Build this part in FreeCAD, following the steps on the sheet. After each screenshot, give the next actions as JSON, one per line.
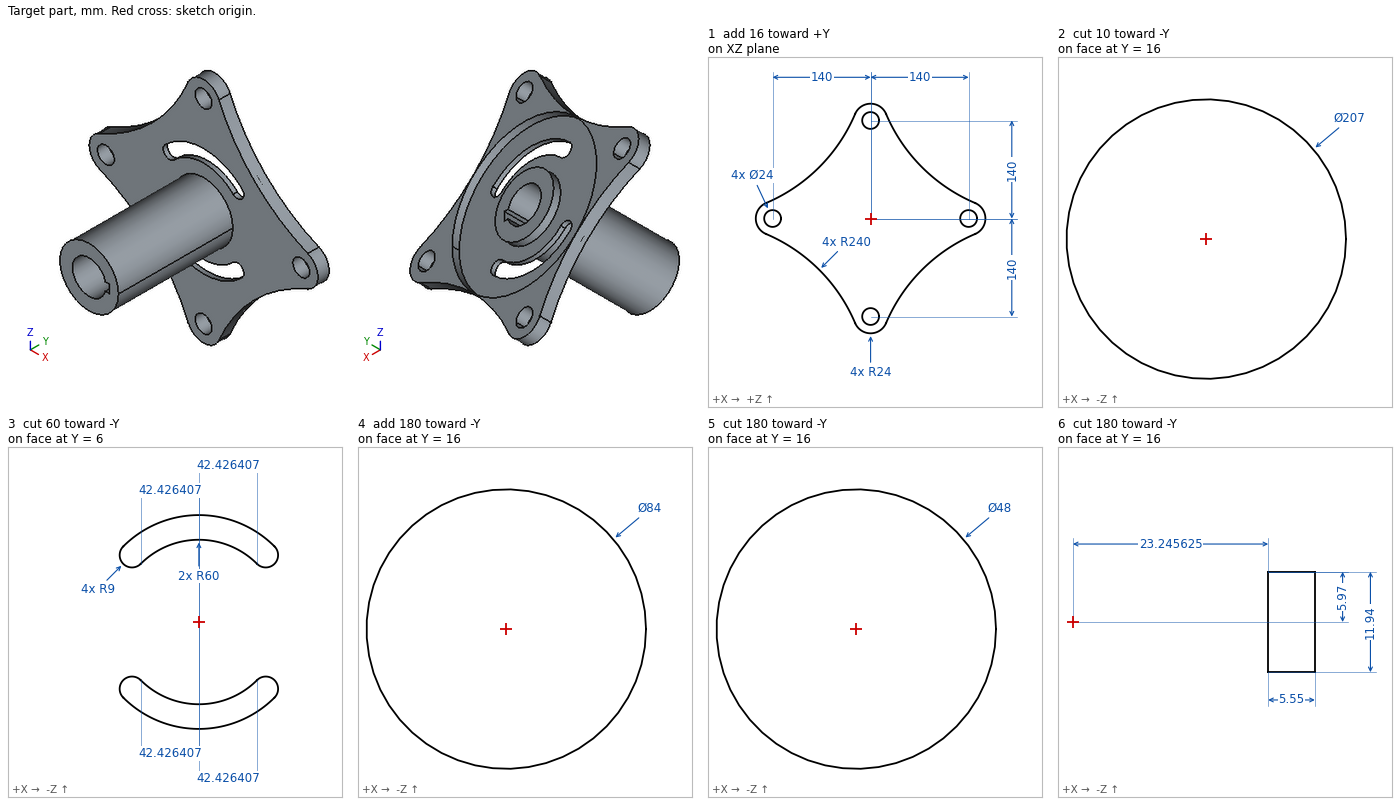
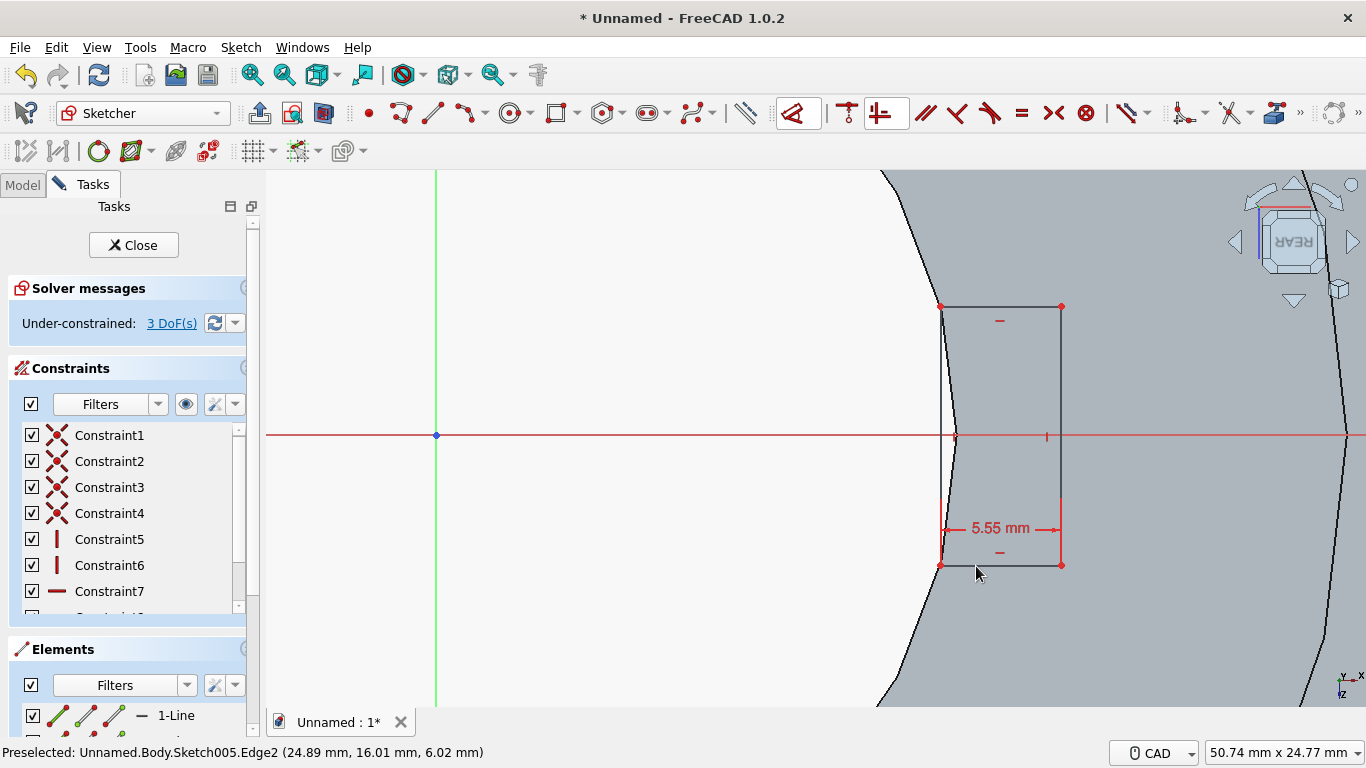
{"action": "left_click", "coordinate": [941, 385]}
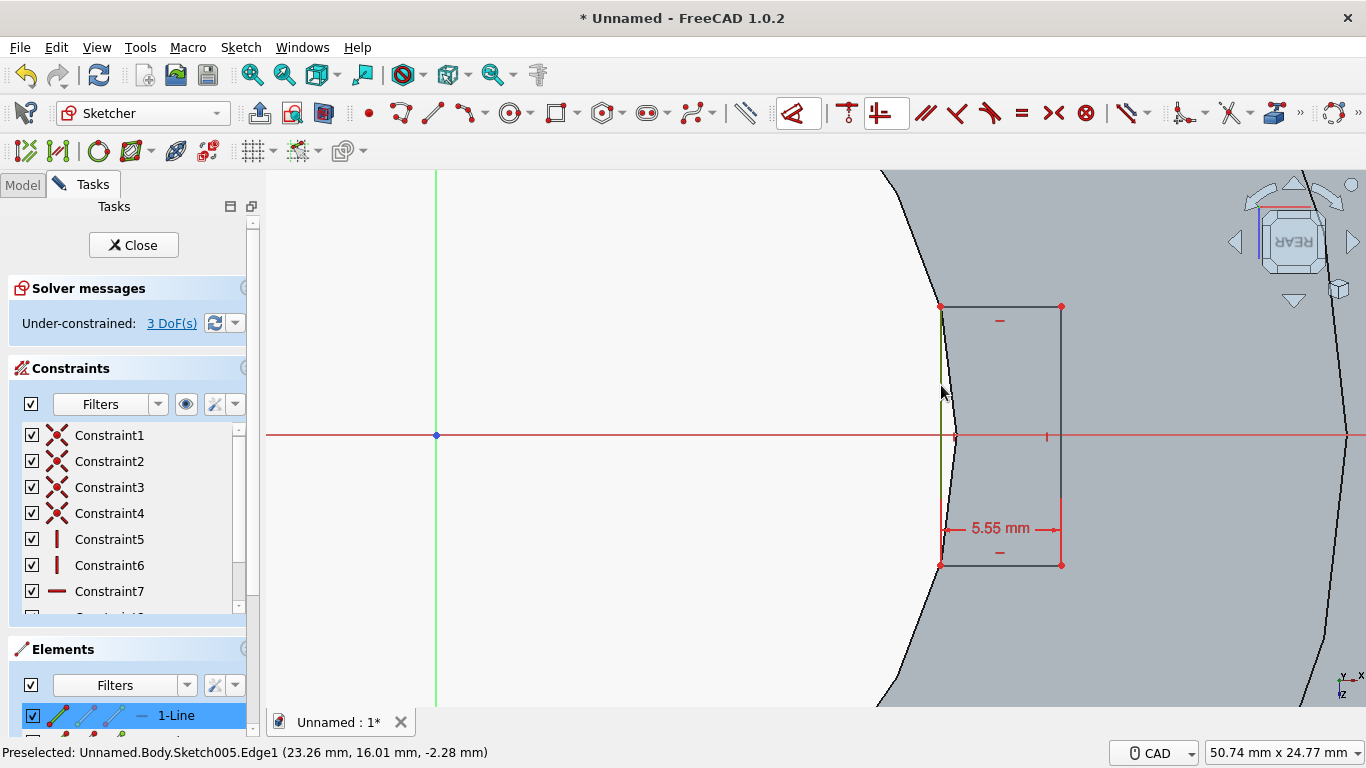
{"action": "key", "text": "i"}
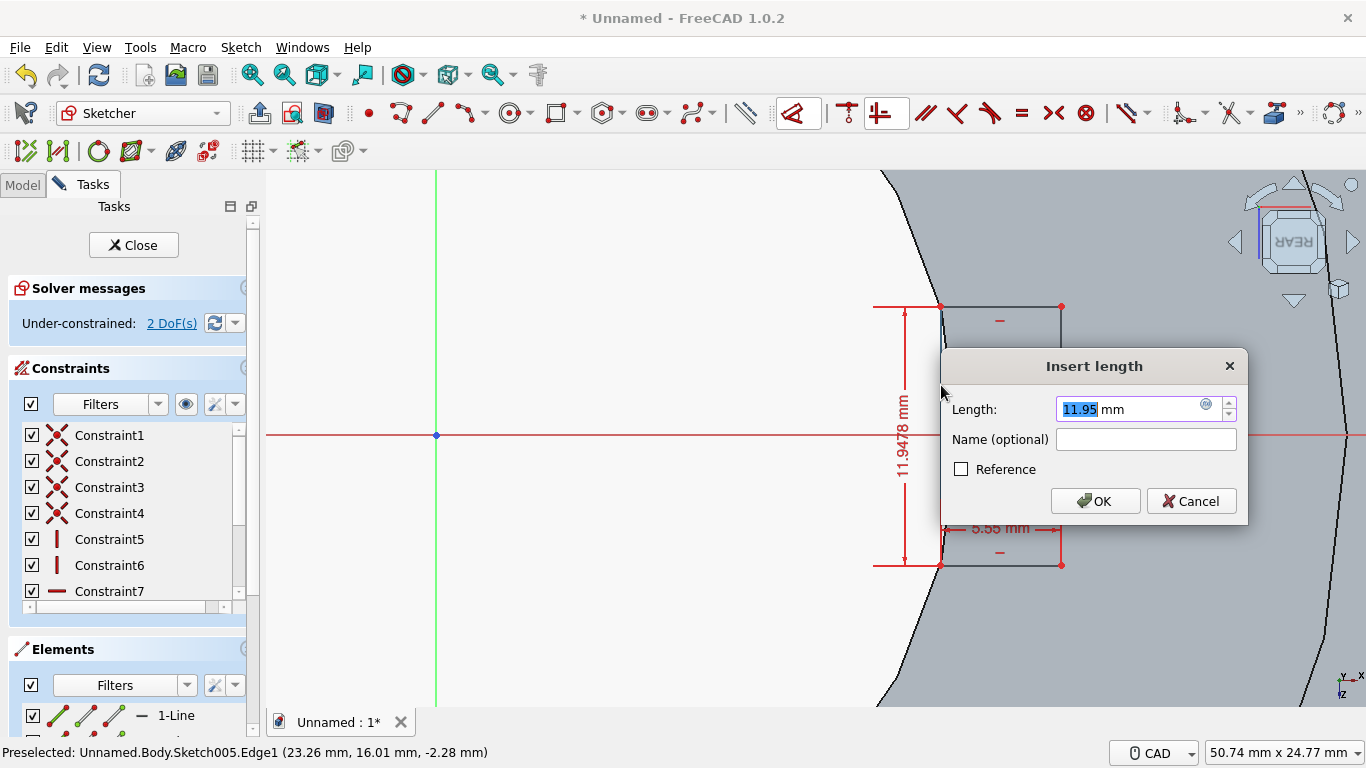
{"action": "type", "text": "11.94"}
{"action": "key", "text": "Return"}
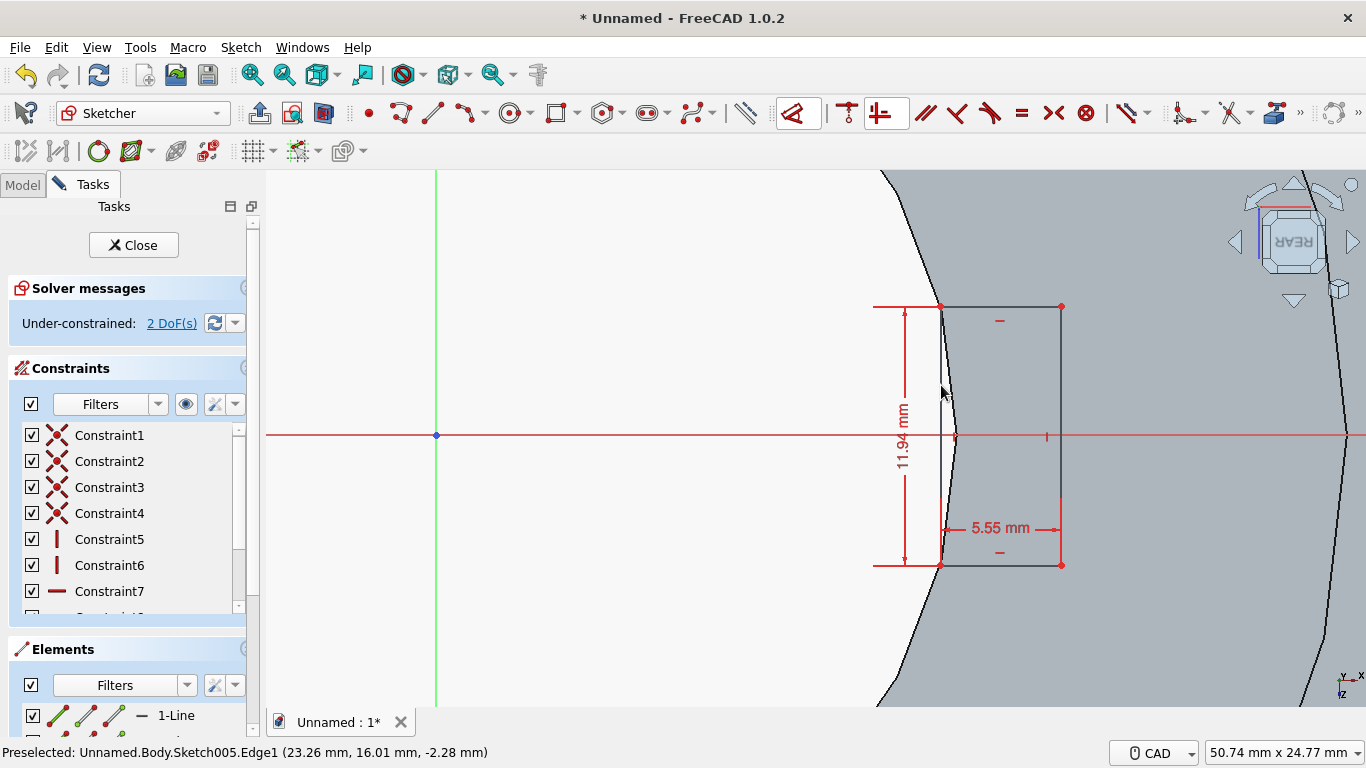
{"action": "left_click", "coordinate": [941, 307]}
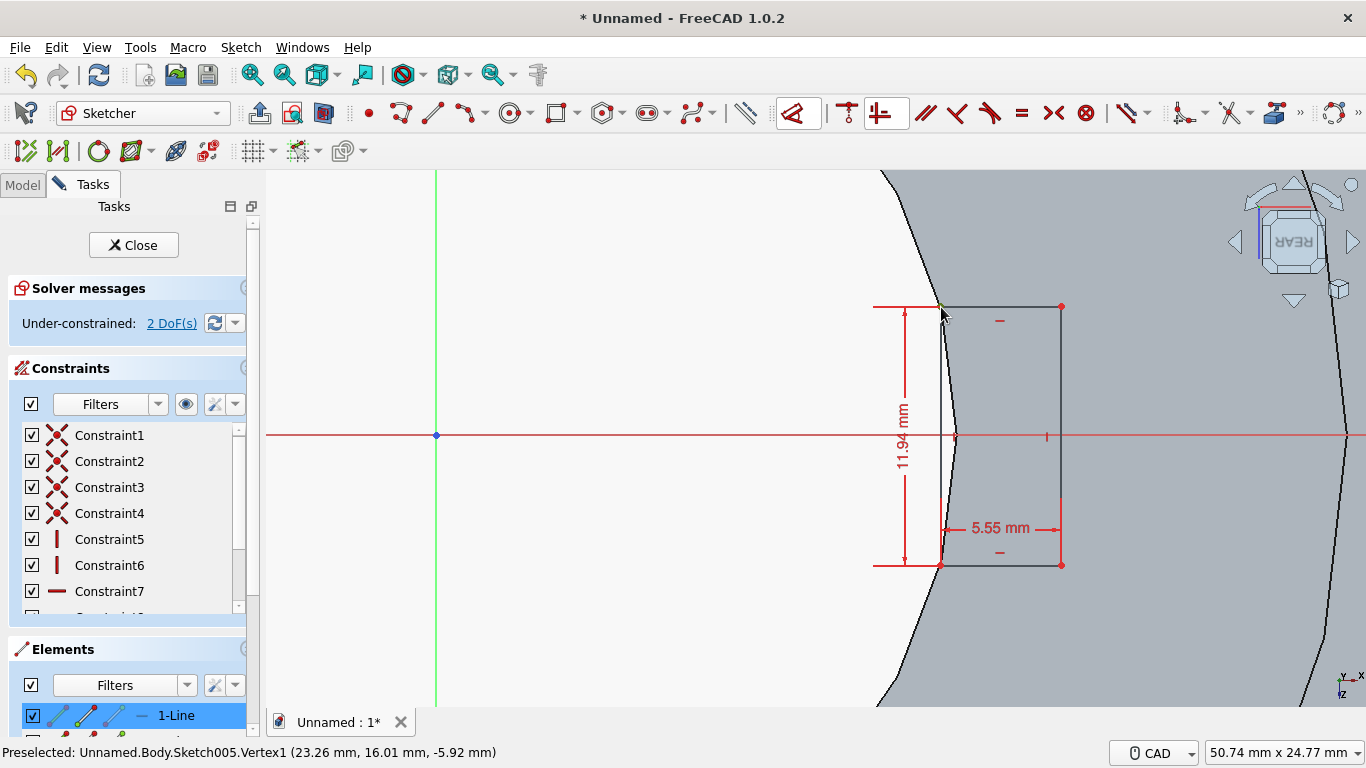
{"action": "key", "text": "i"}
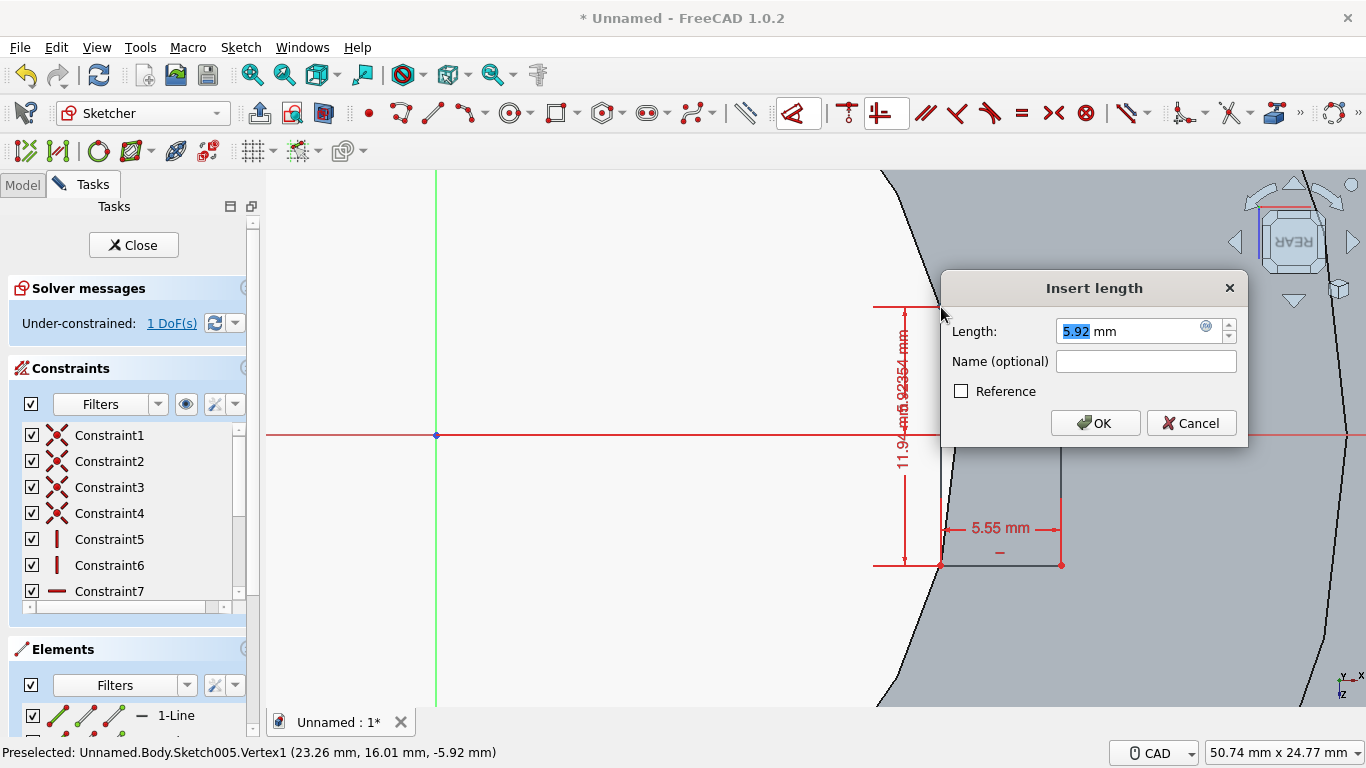
{"action": "type", "text": "5.97"}
{"action": "key", "text": "Return"}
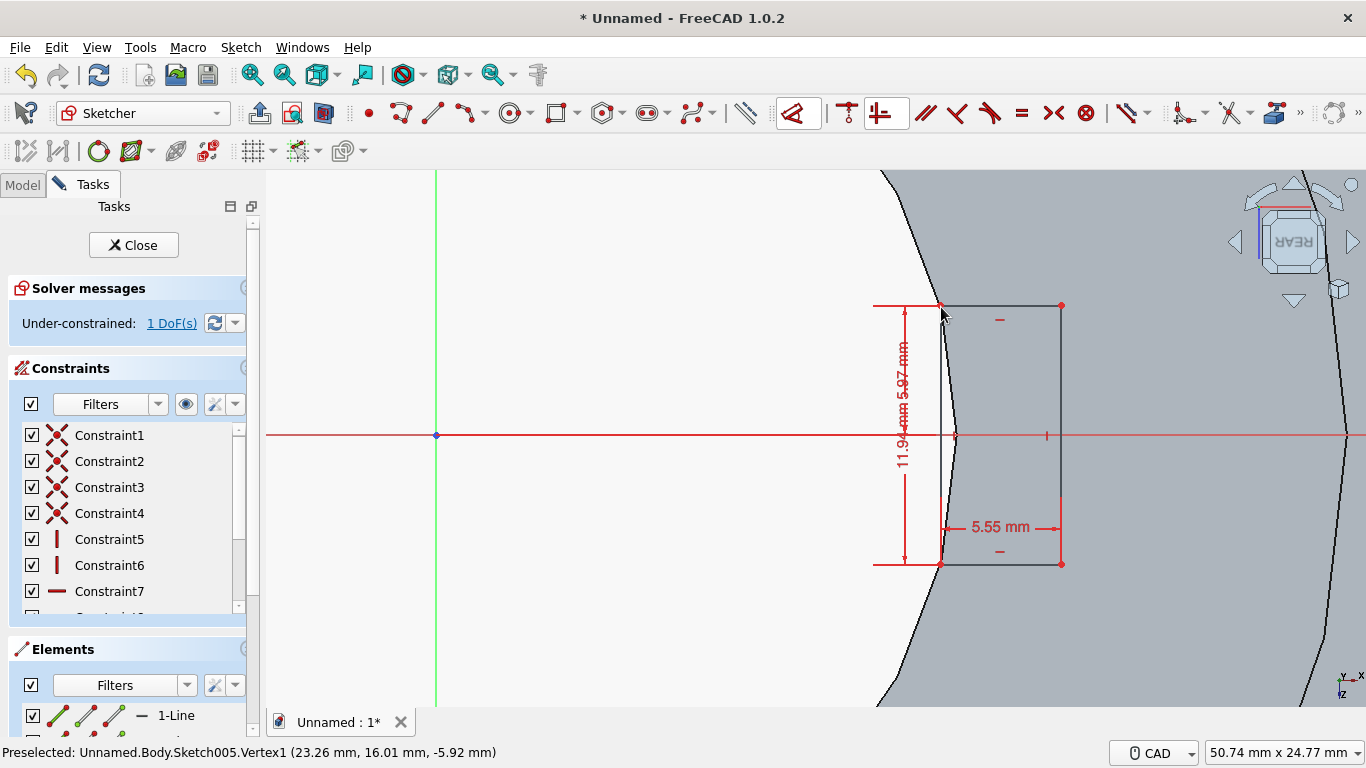
{"action": "left_click", "coordinate": [941, 306]}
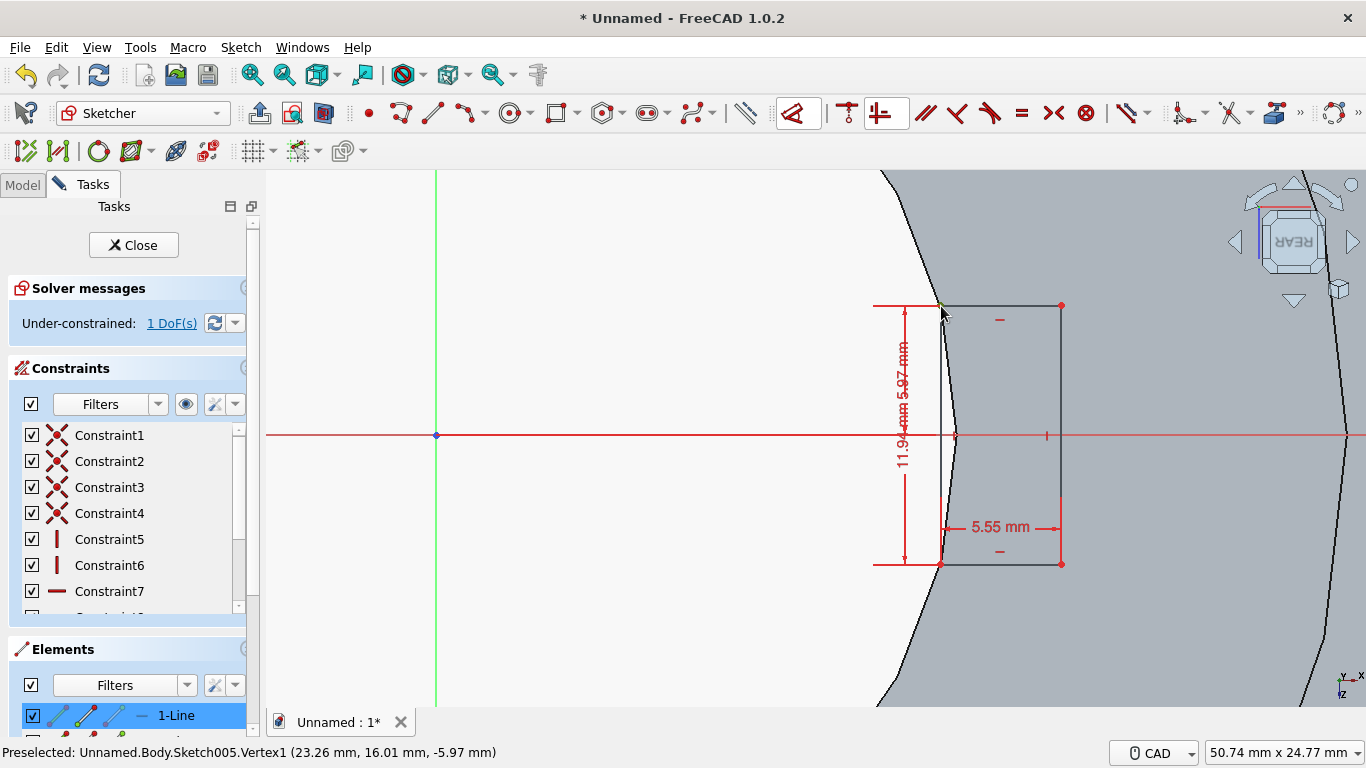
{"action": "left_click", "coordinate": [816, 114]}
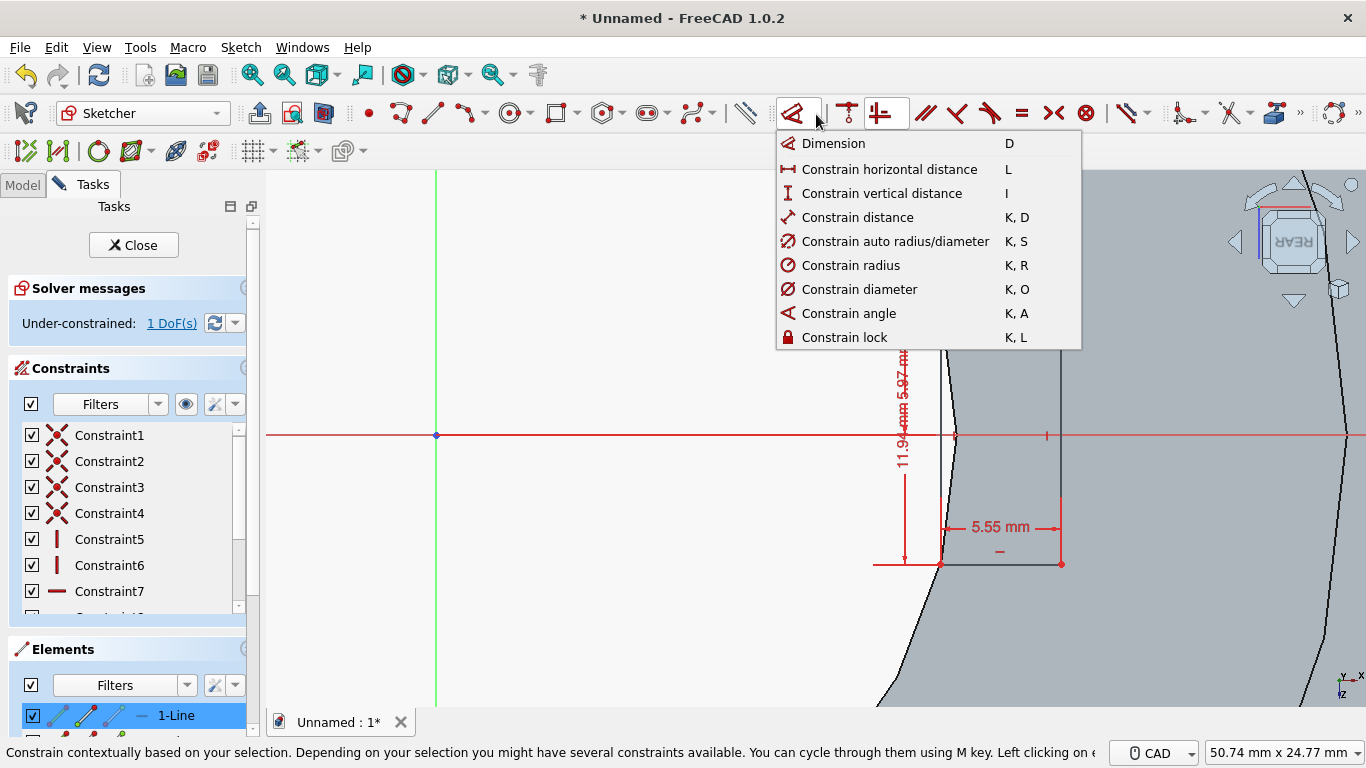
{"action": "left_click", "coordinate": [929, 169]}